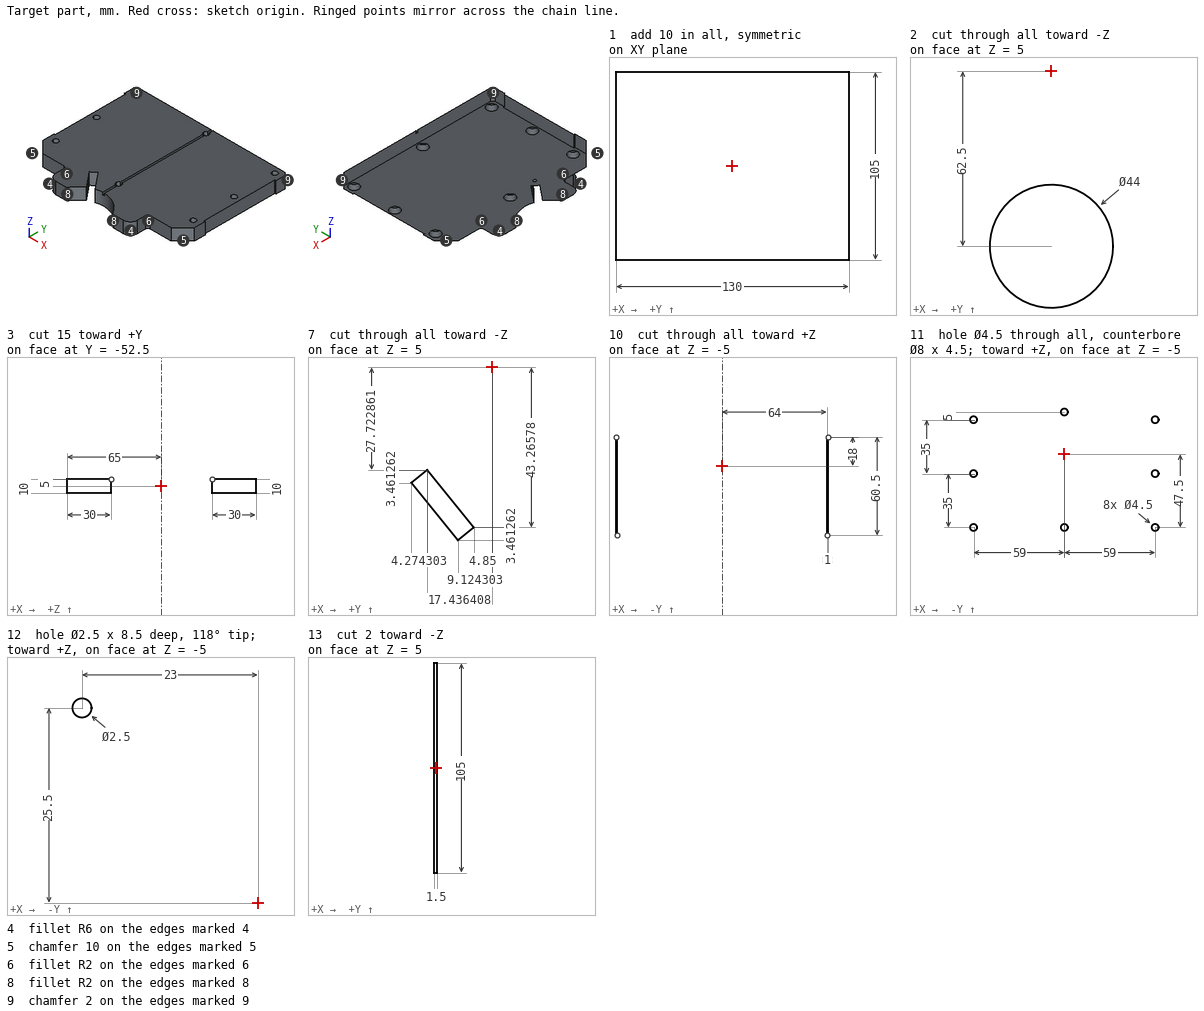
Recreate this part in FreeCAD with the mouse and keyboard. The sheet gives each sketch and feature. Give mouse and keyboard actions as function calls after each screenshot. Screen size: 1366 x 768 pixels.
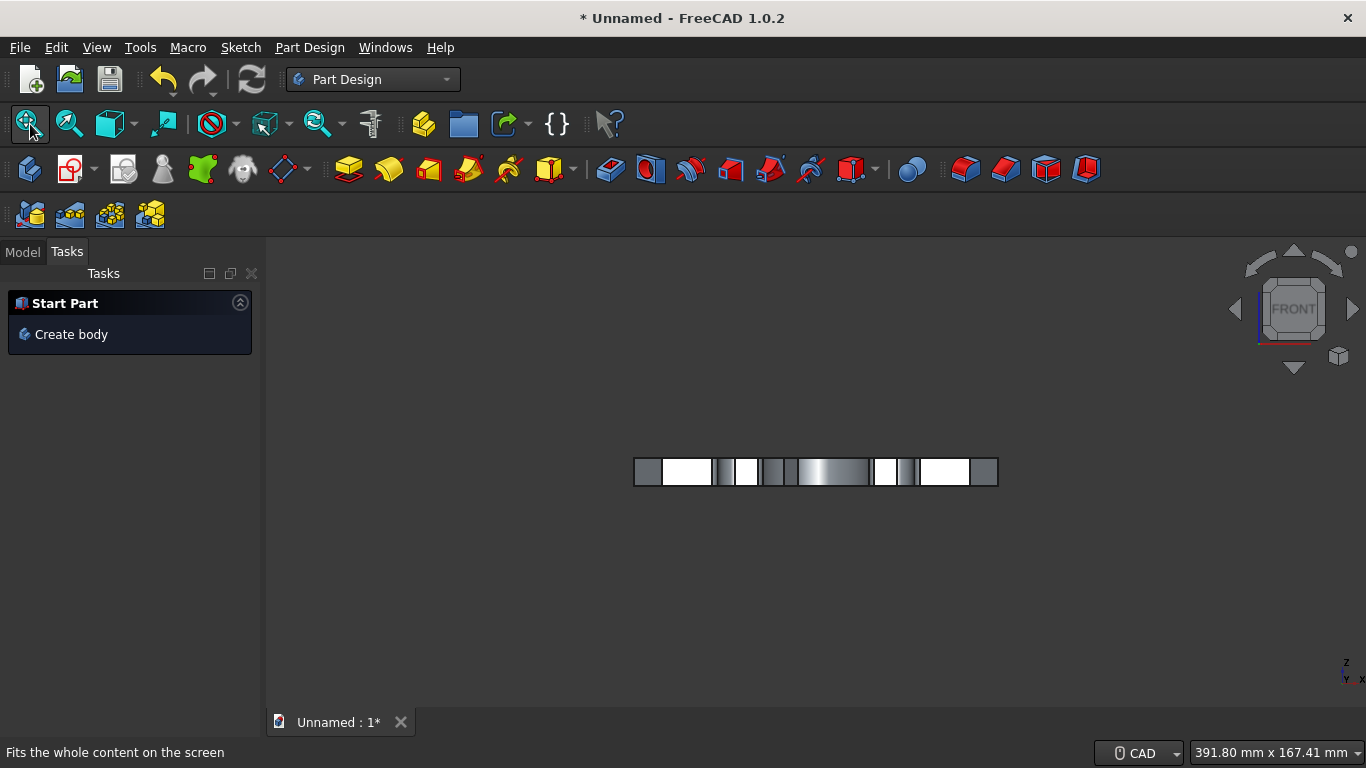
click(30, 124)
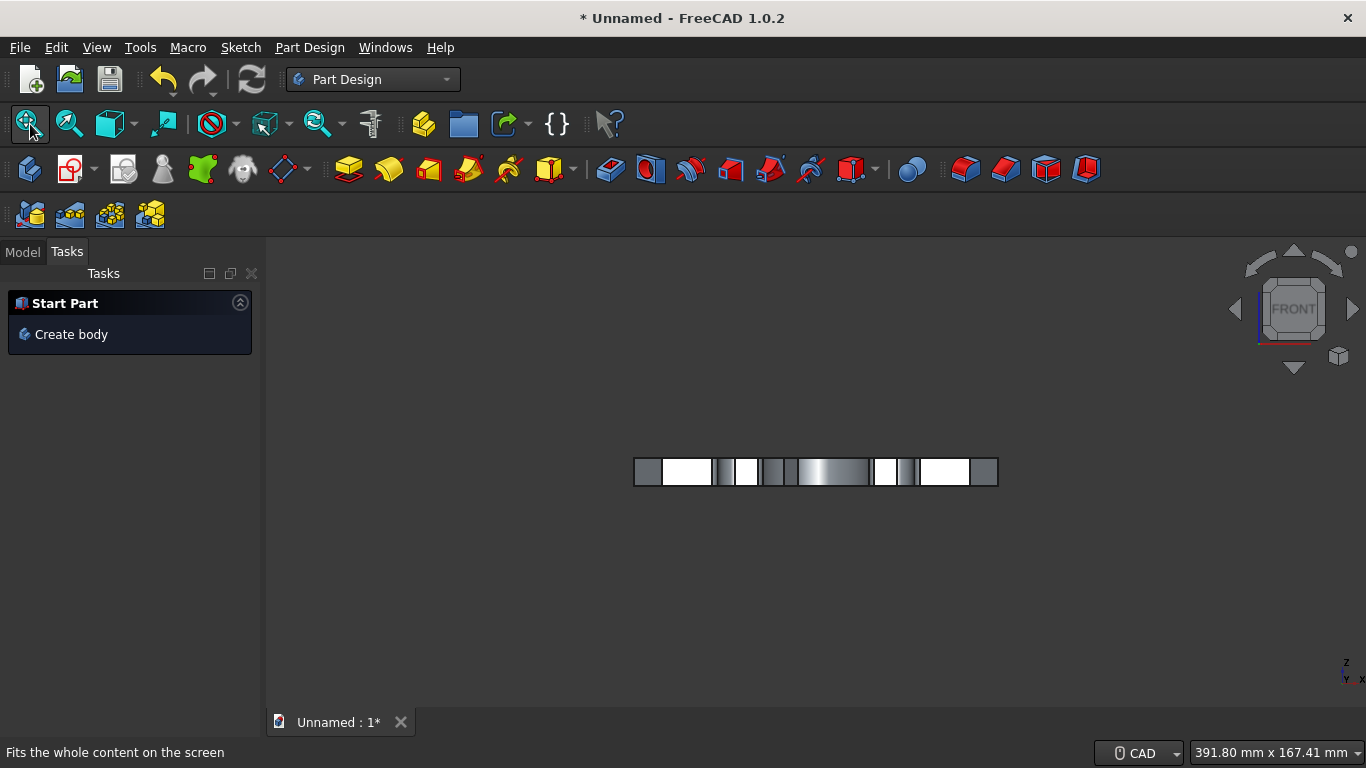
key(3)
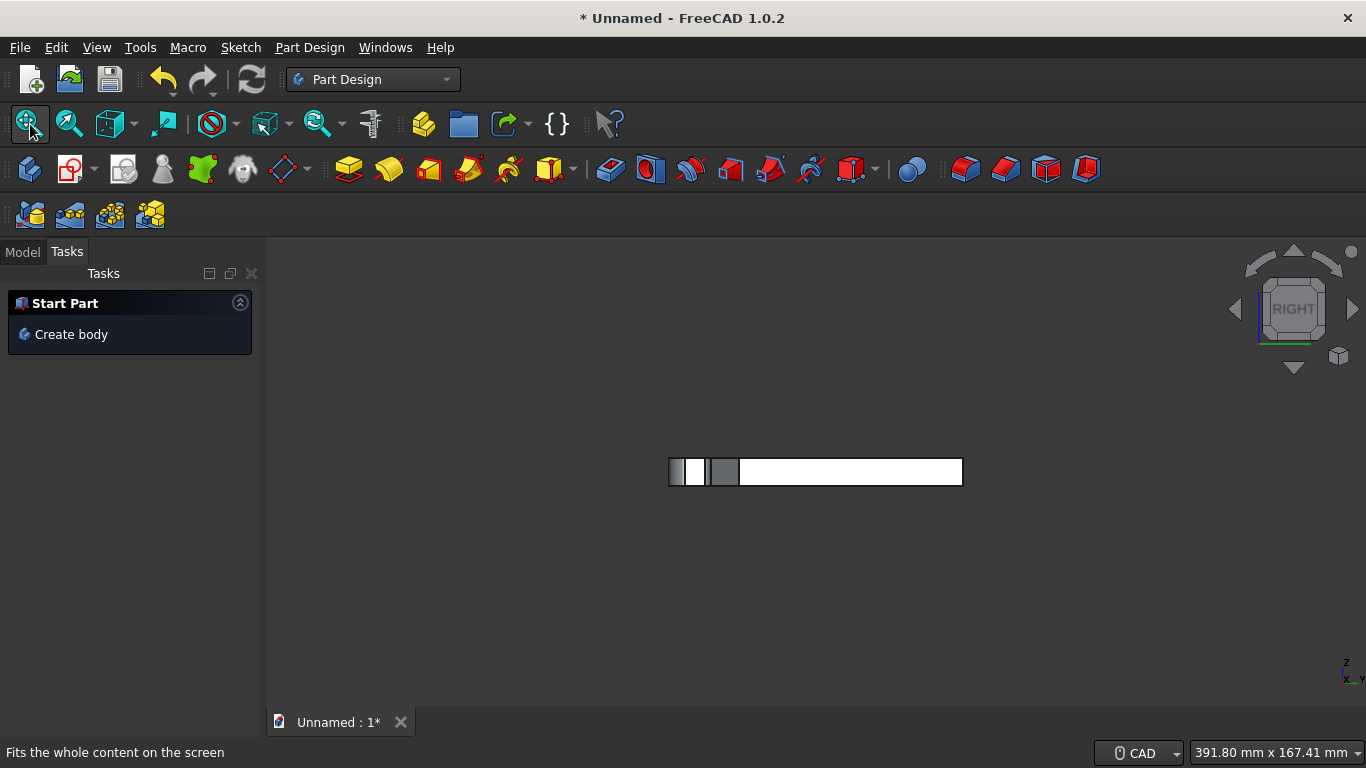
click(30, 124)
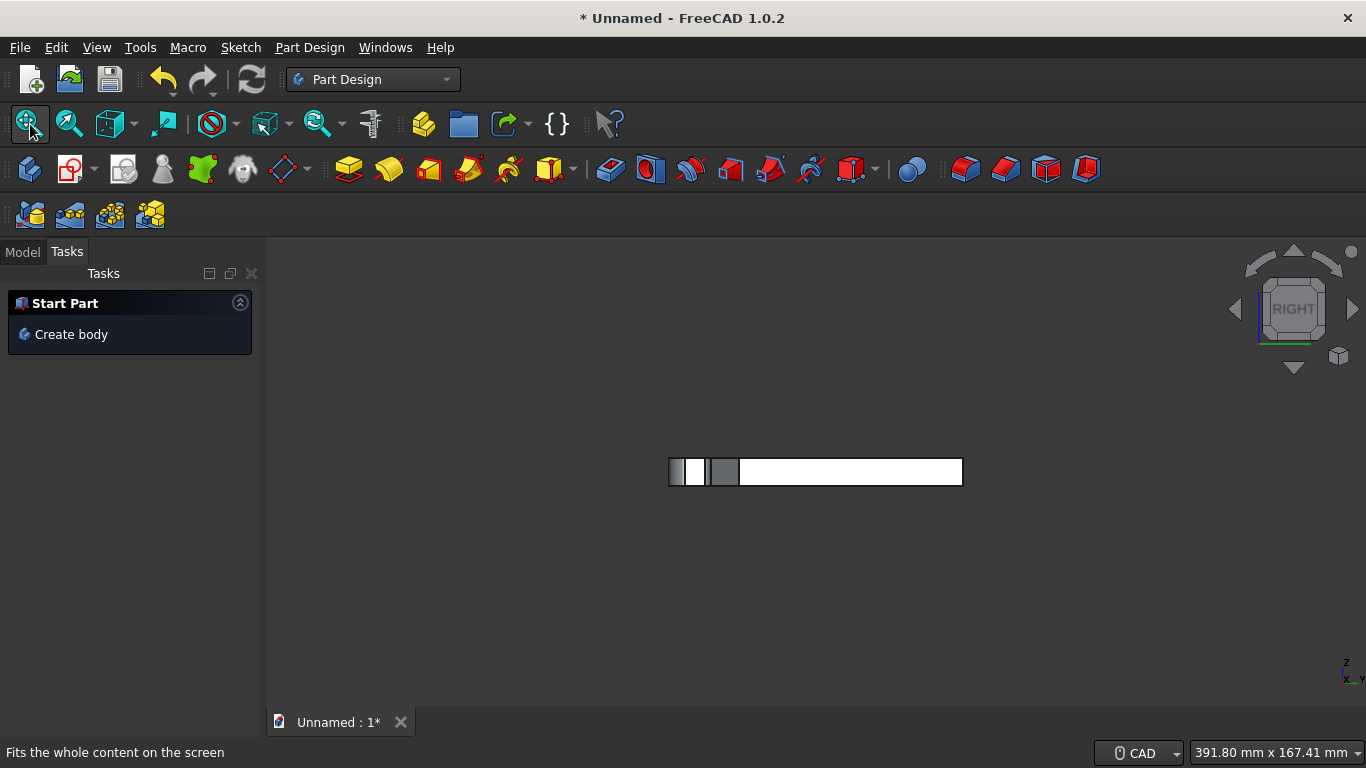
click(963, 471)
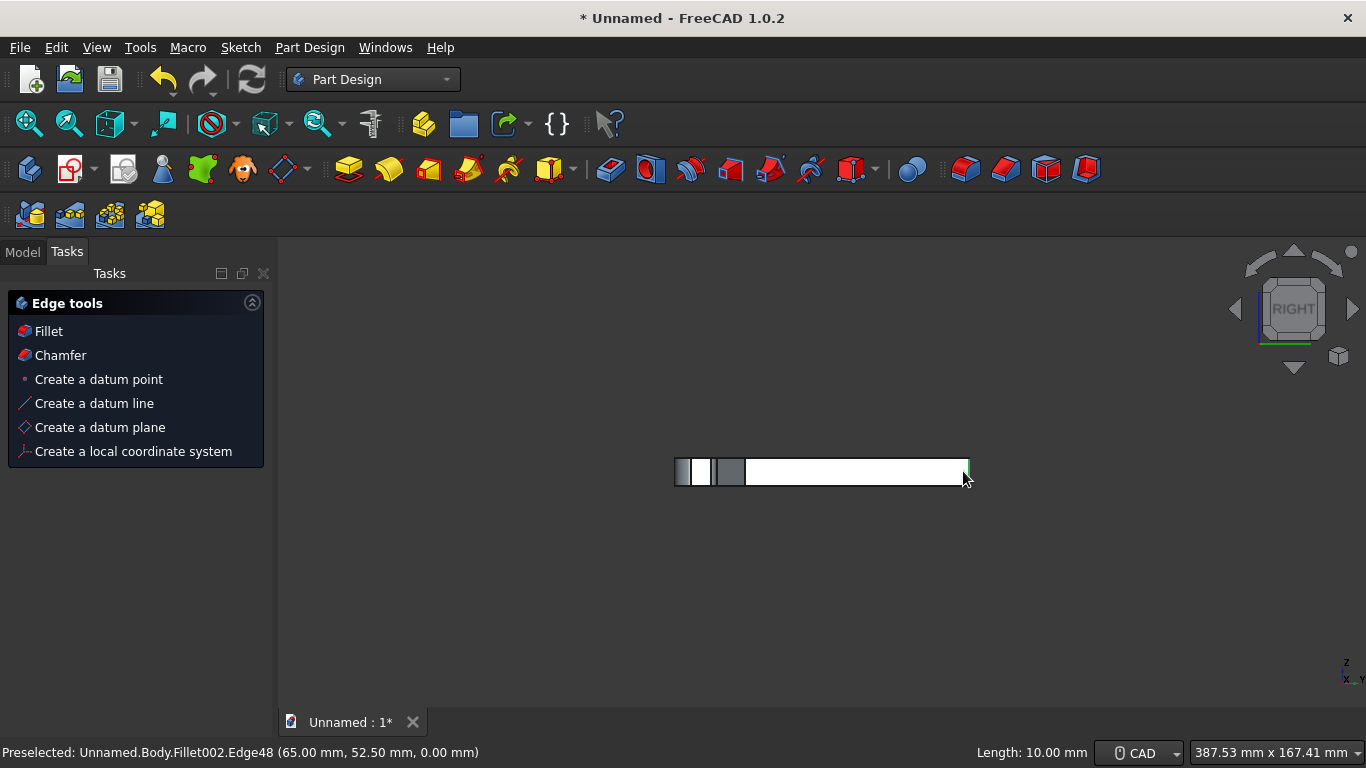
key(5)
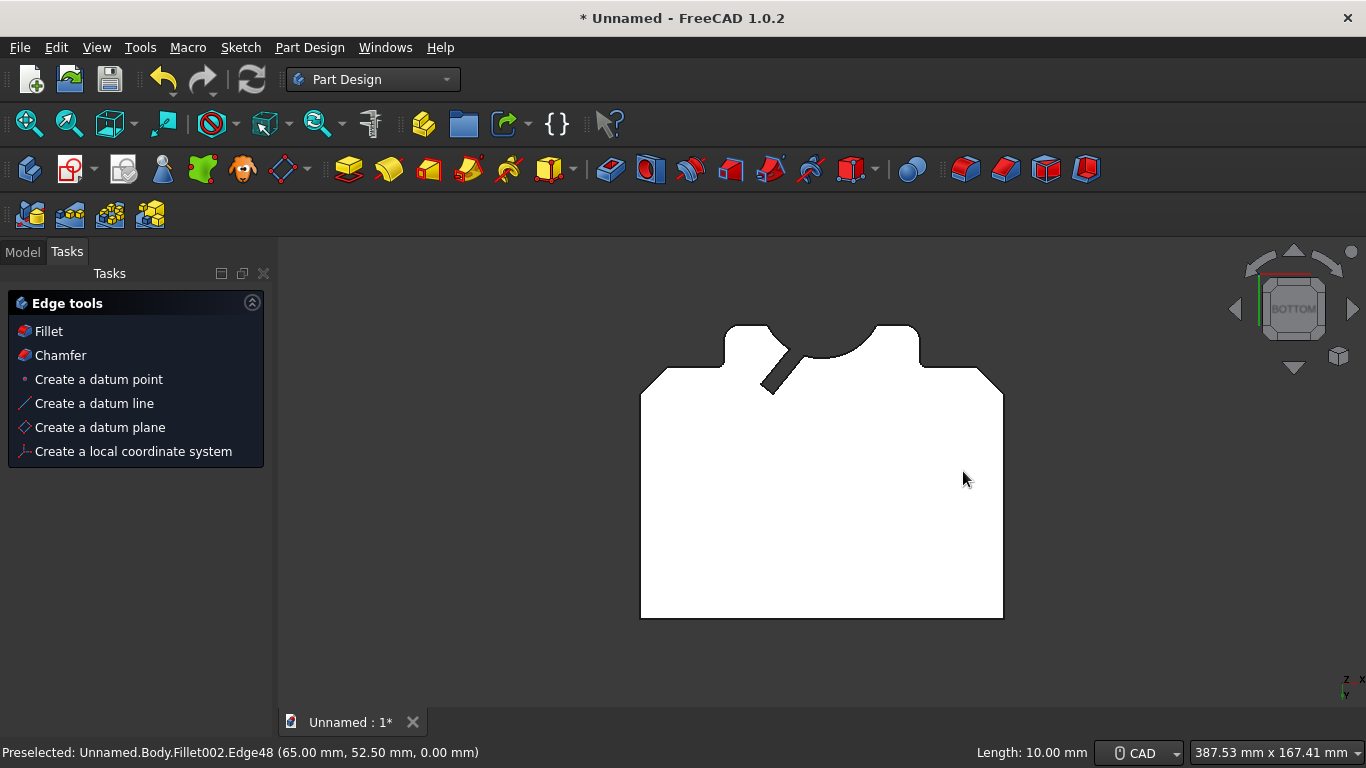
key(4)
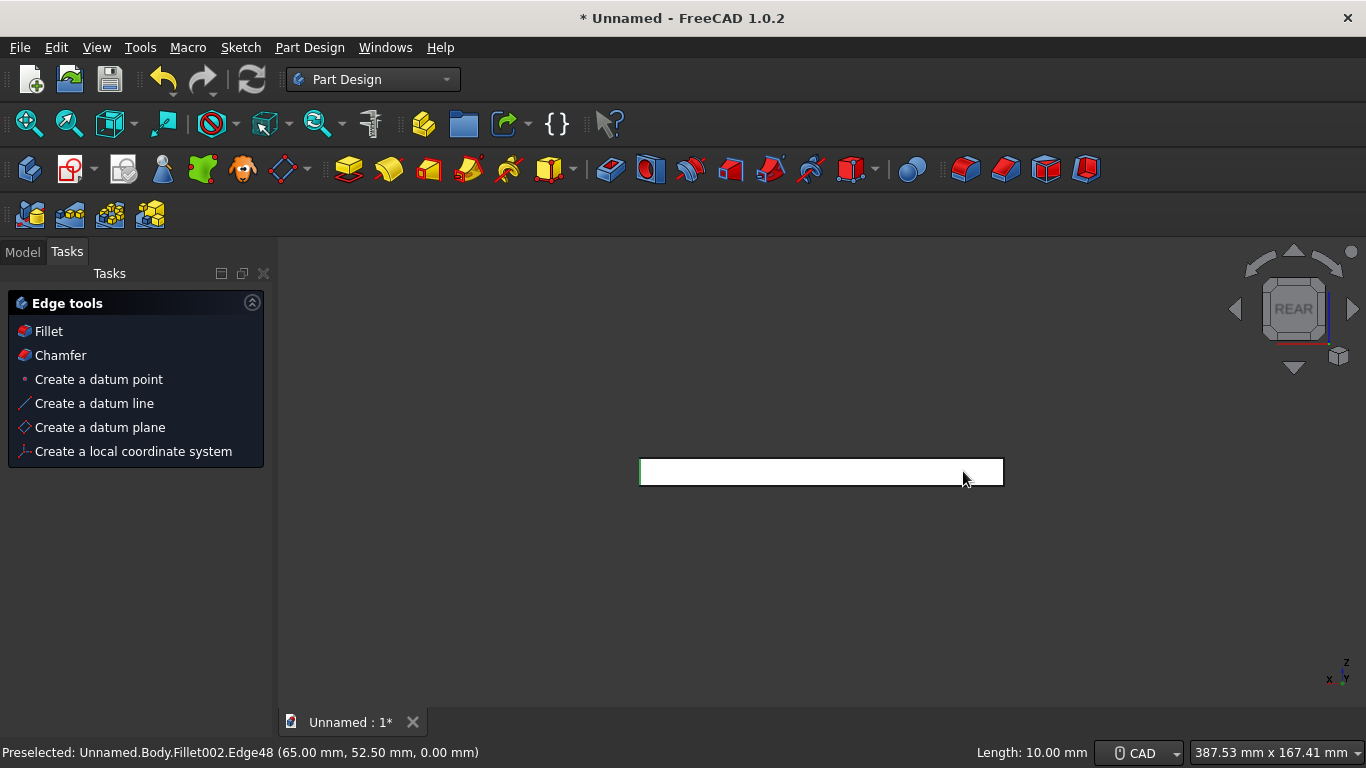
click(30, 124)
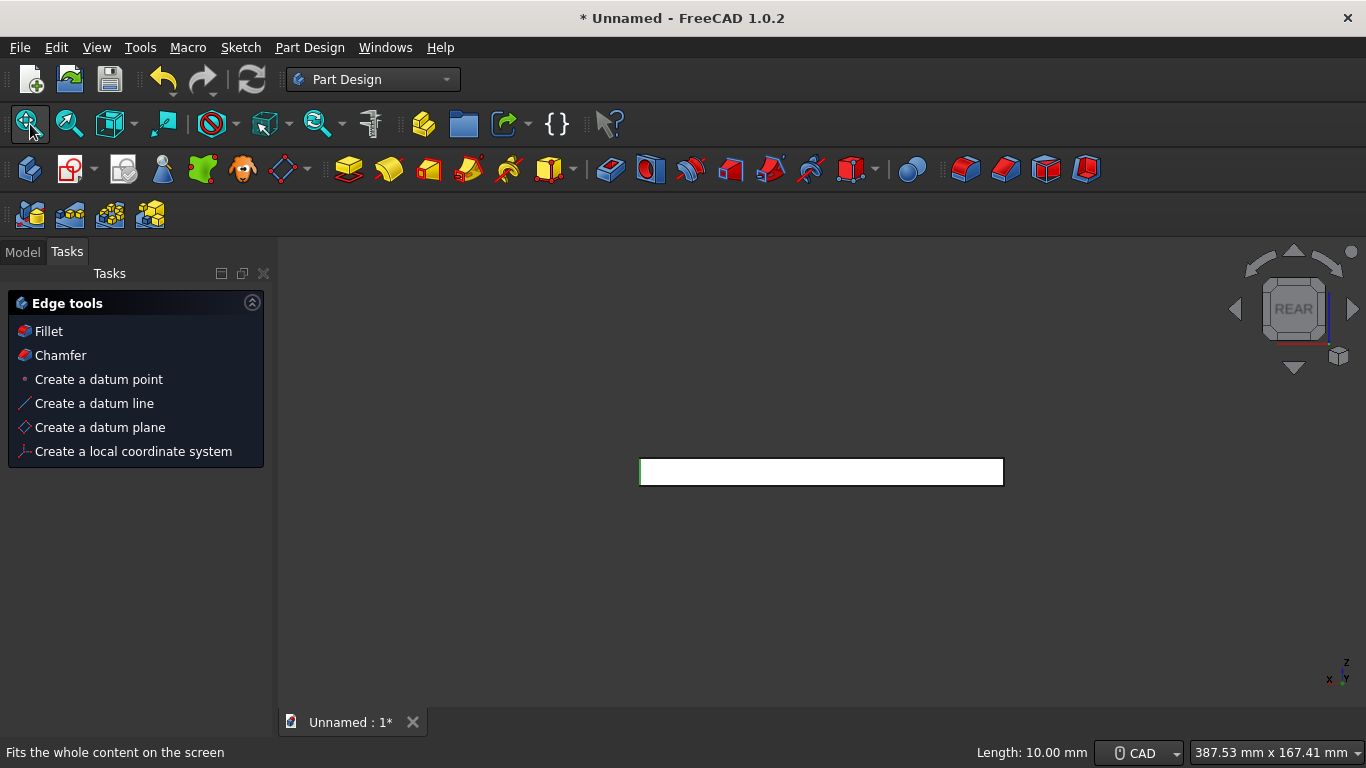
click(1004, 471, ctrl)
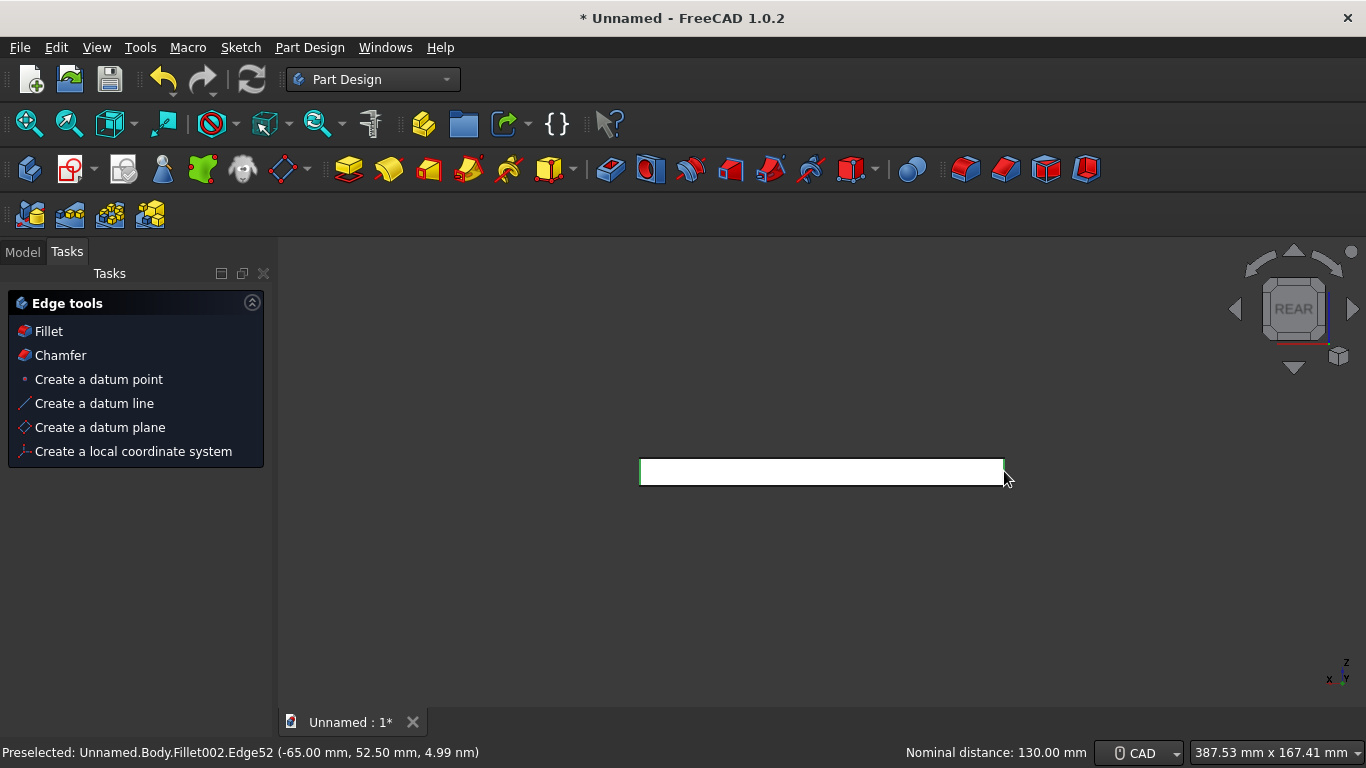
click(1006, 170)